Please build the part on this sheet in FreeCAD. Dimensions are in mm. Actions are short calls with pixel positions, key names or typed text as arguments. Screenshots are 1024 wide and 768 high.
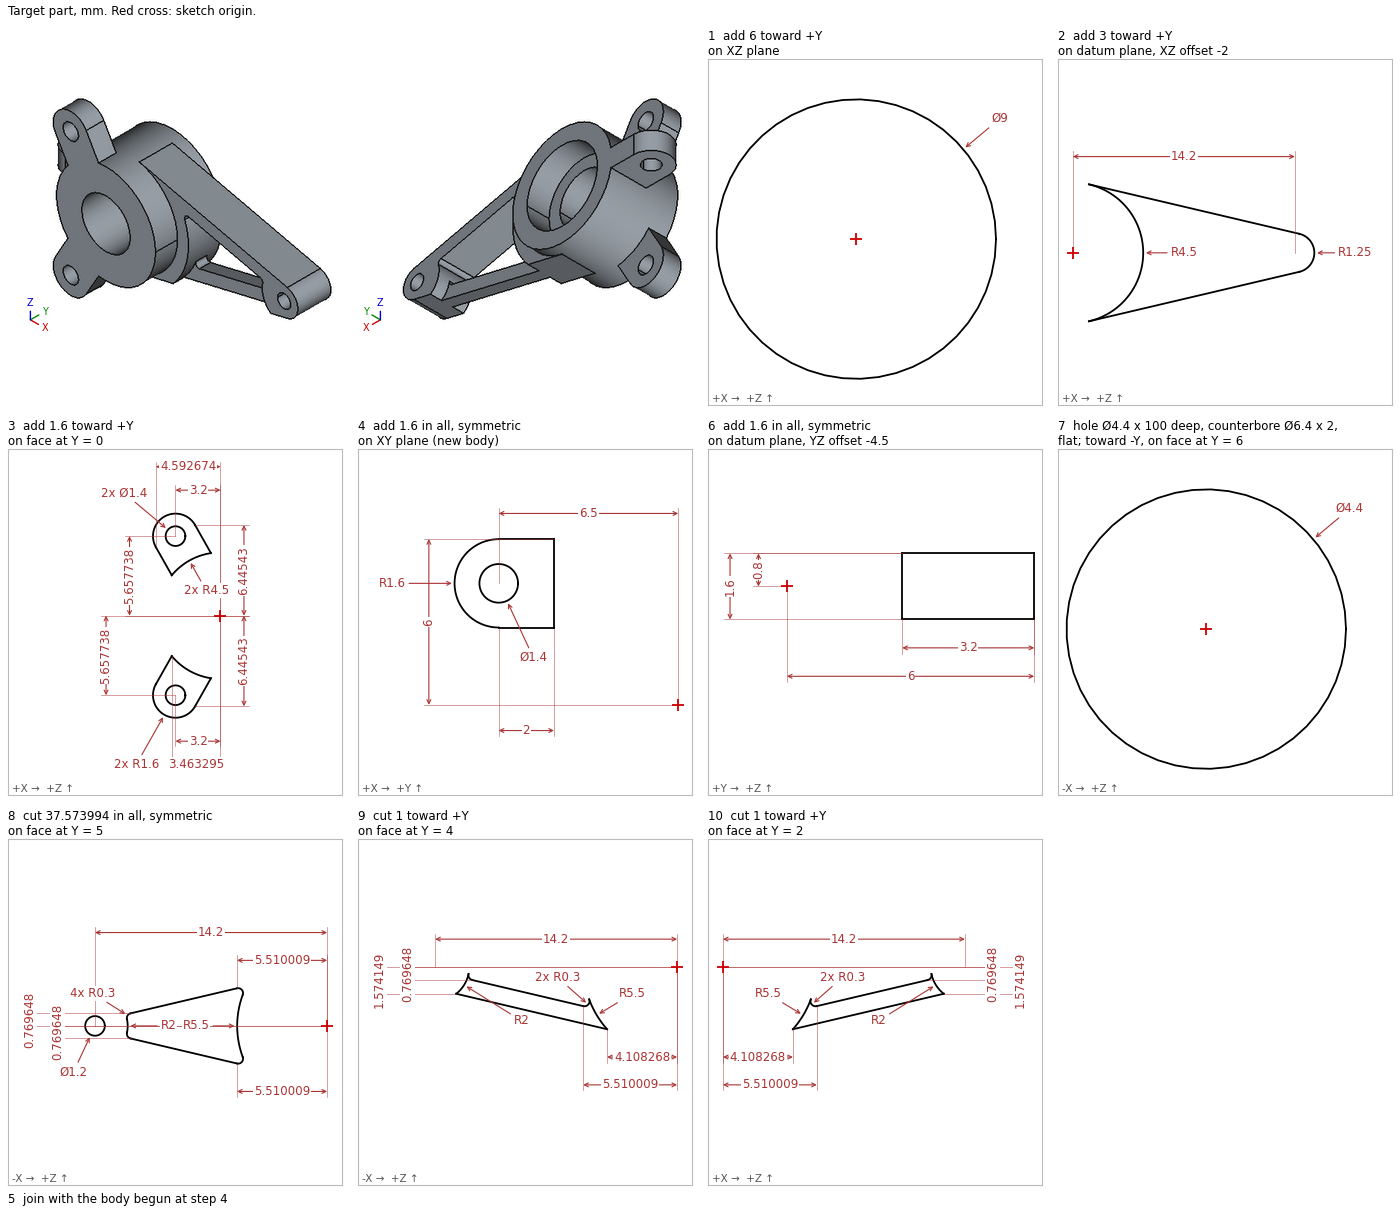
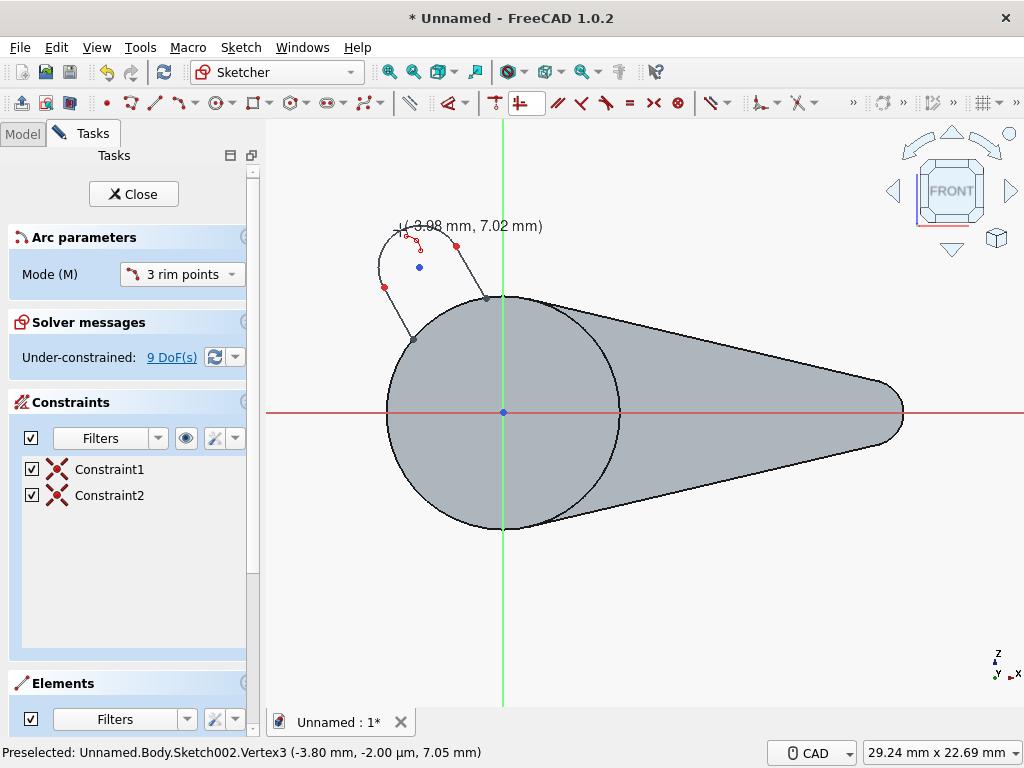
click(413, 340)
click(486, 299)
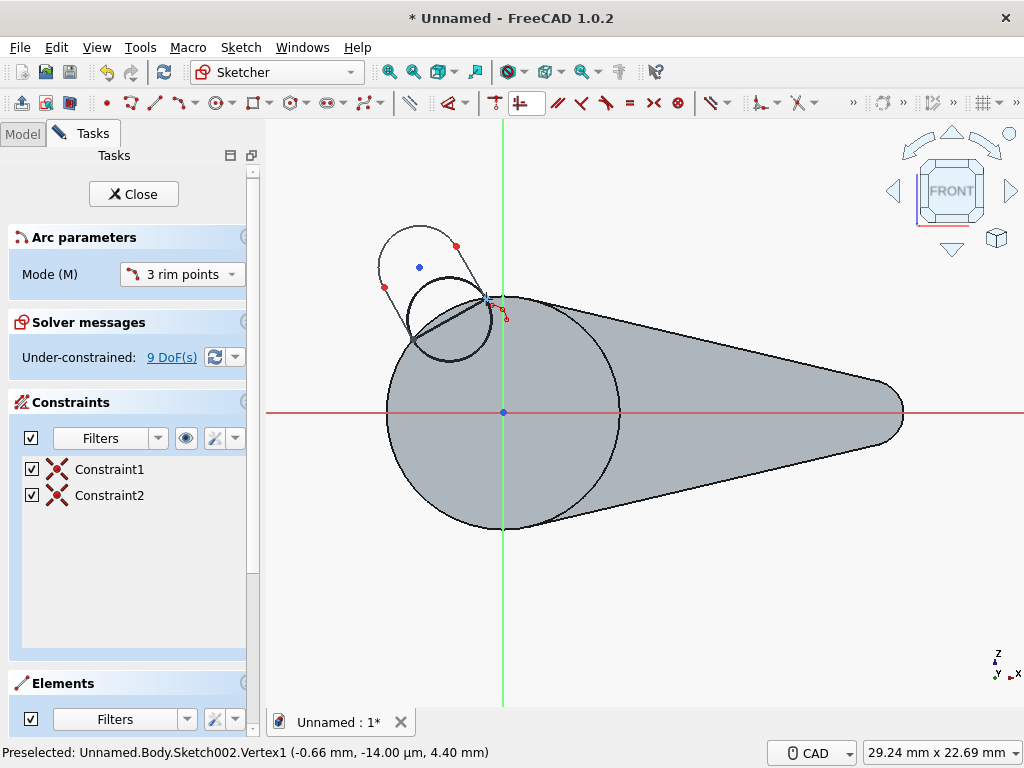
scroll(446, 311, up, 4)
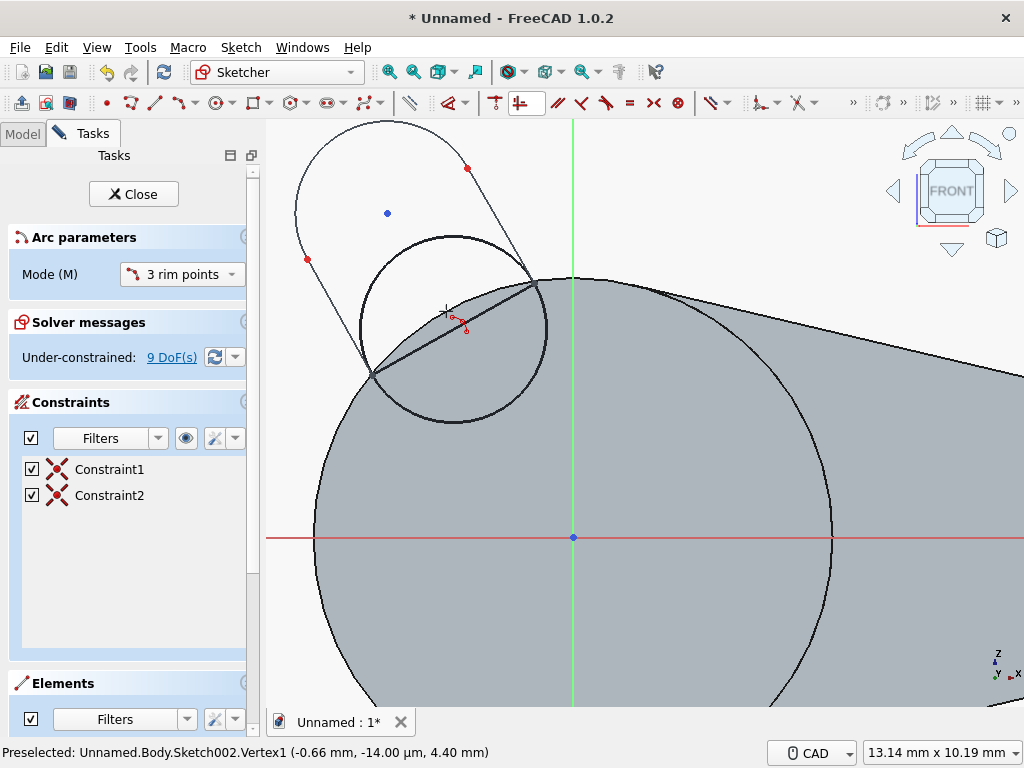
click(445, 312)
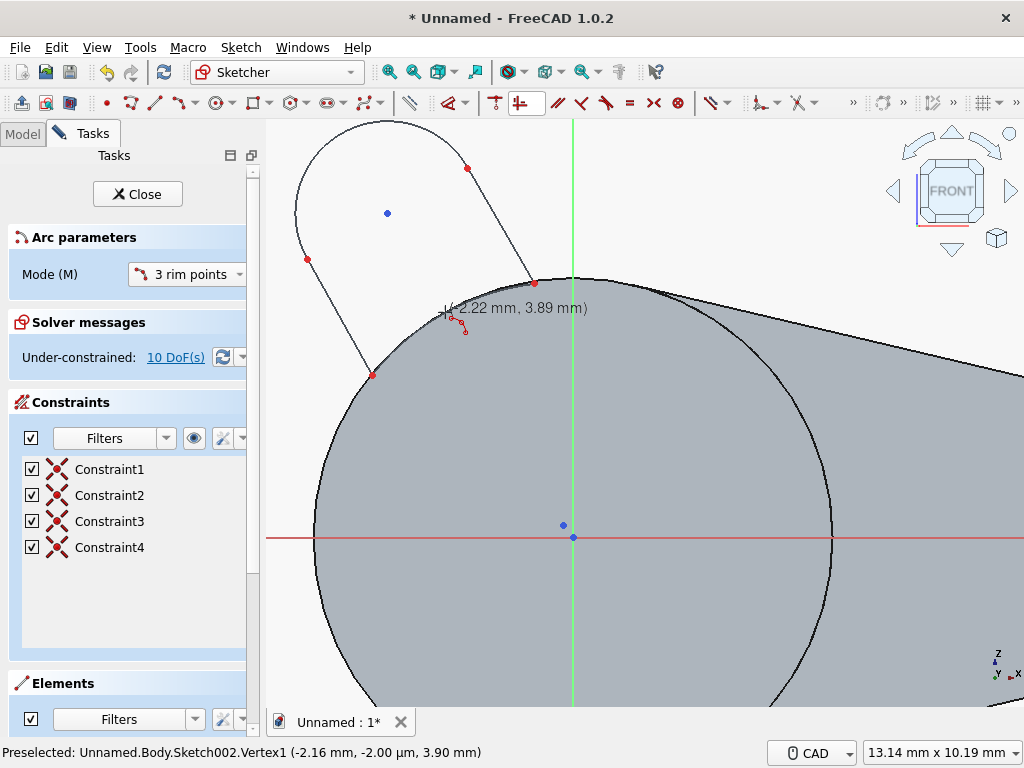
click(156, 104)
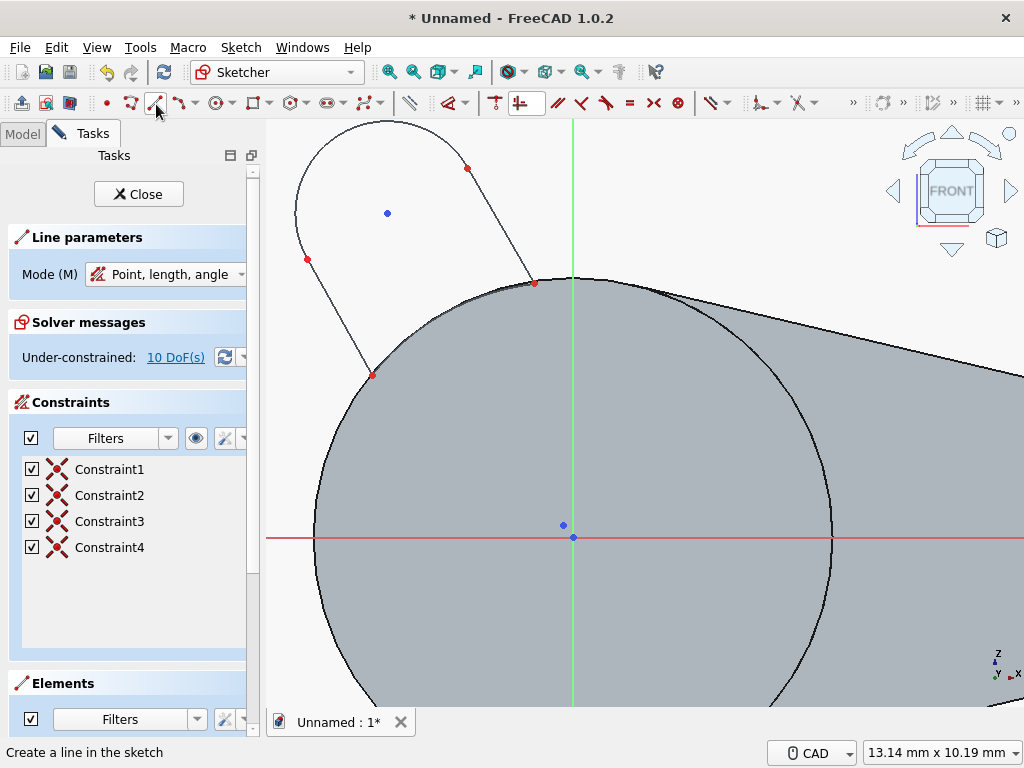
scroll(687, 311, down, 4)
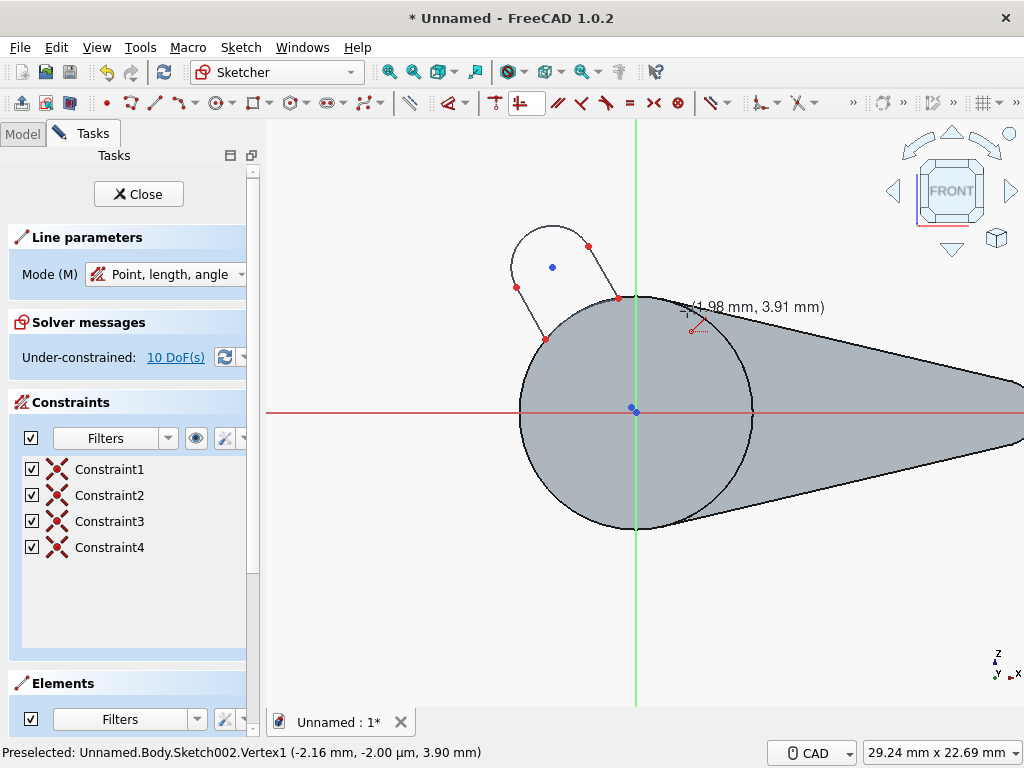
click(589, 580)
click(619, 528)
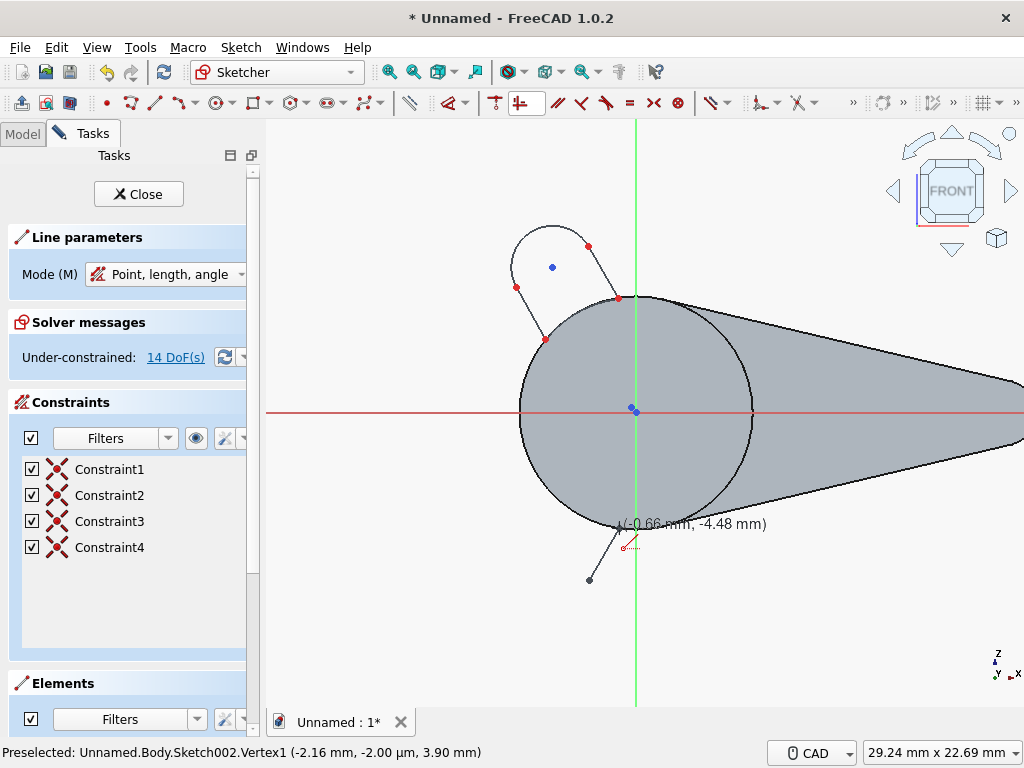
click(546, 487)
click(517, 539)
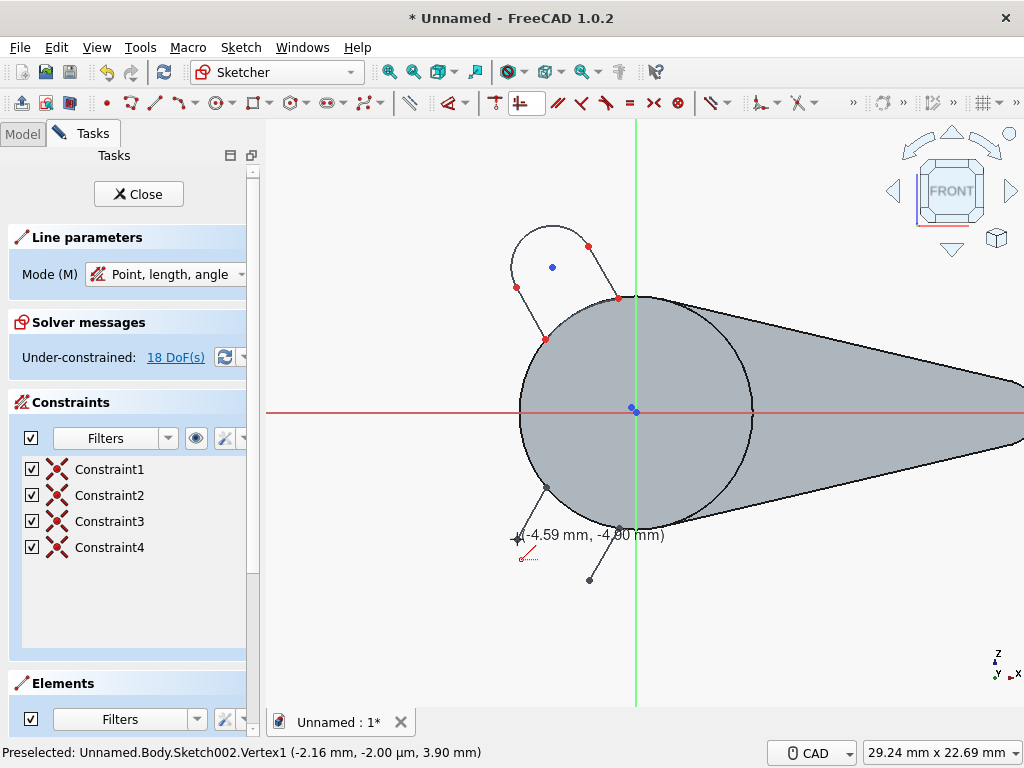
key(g)
key(3)
key(a)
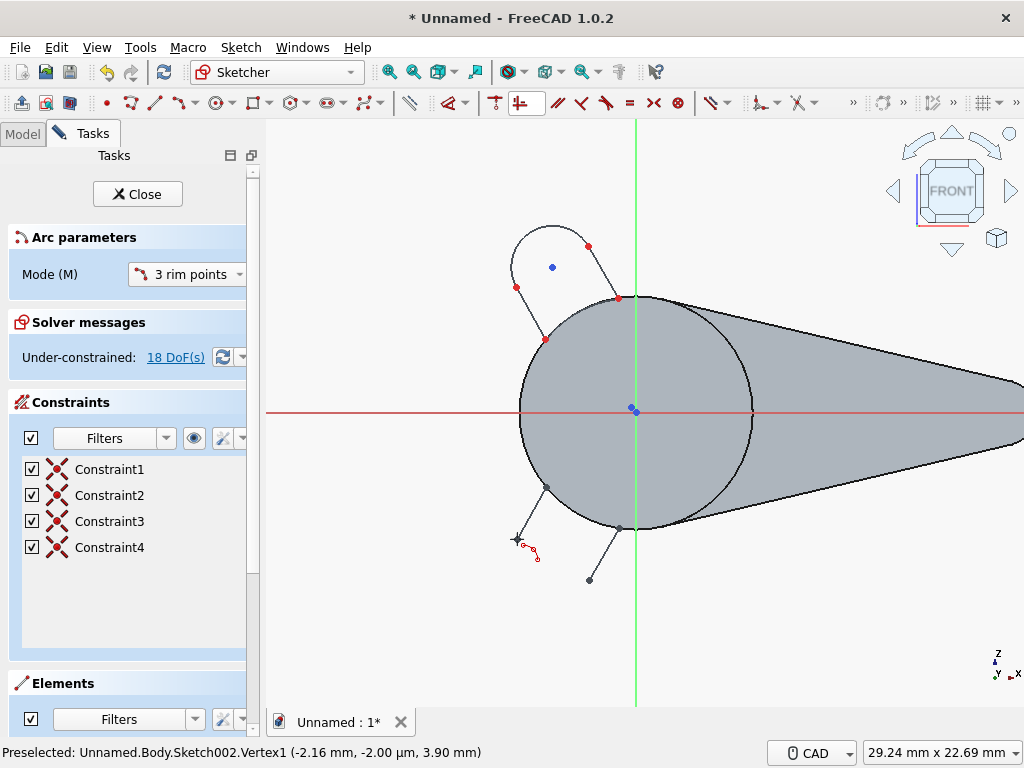
click(619, 529)
click(546, 488)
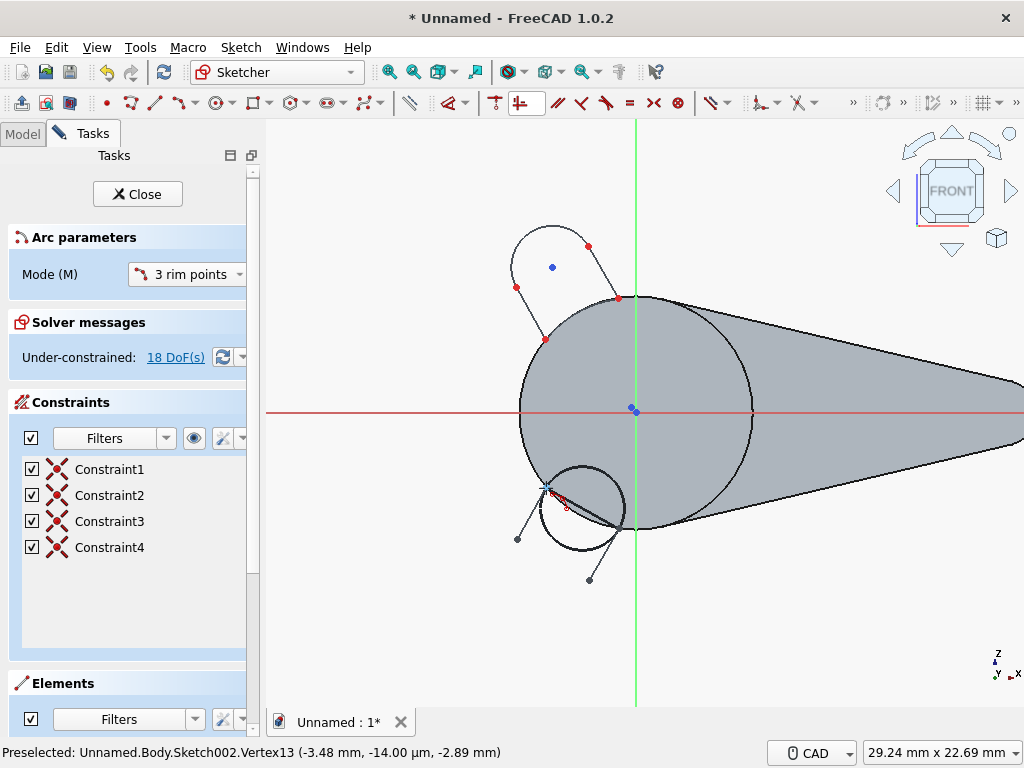
scroll(579, 515, up, 4)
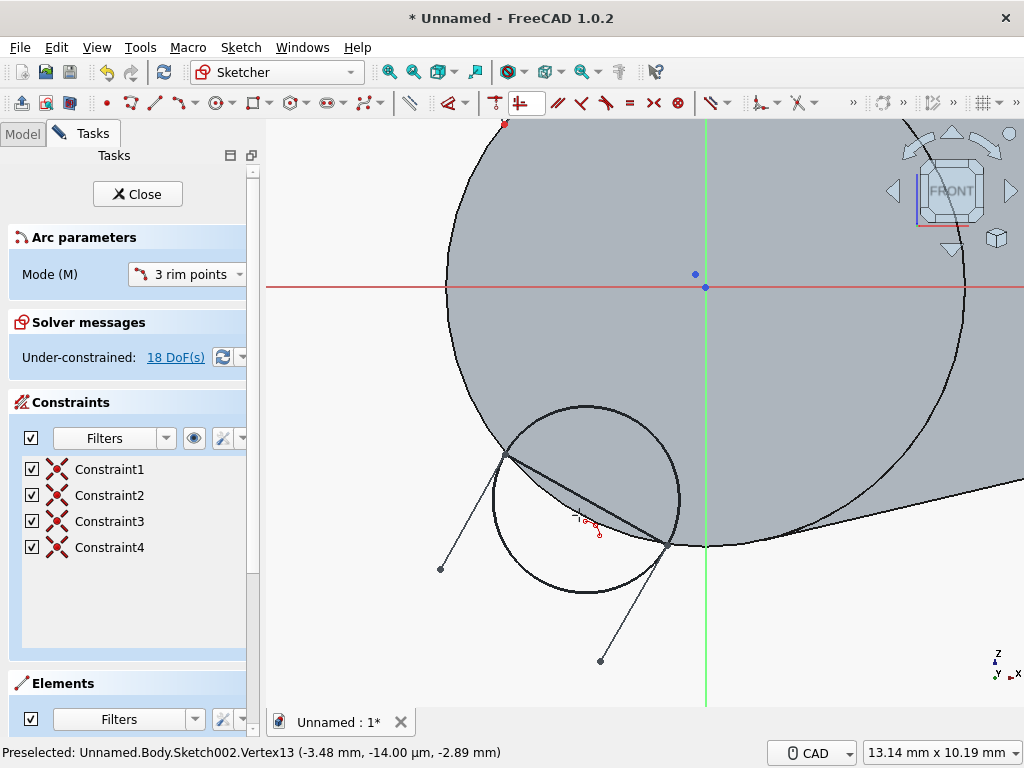
click(578, 513)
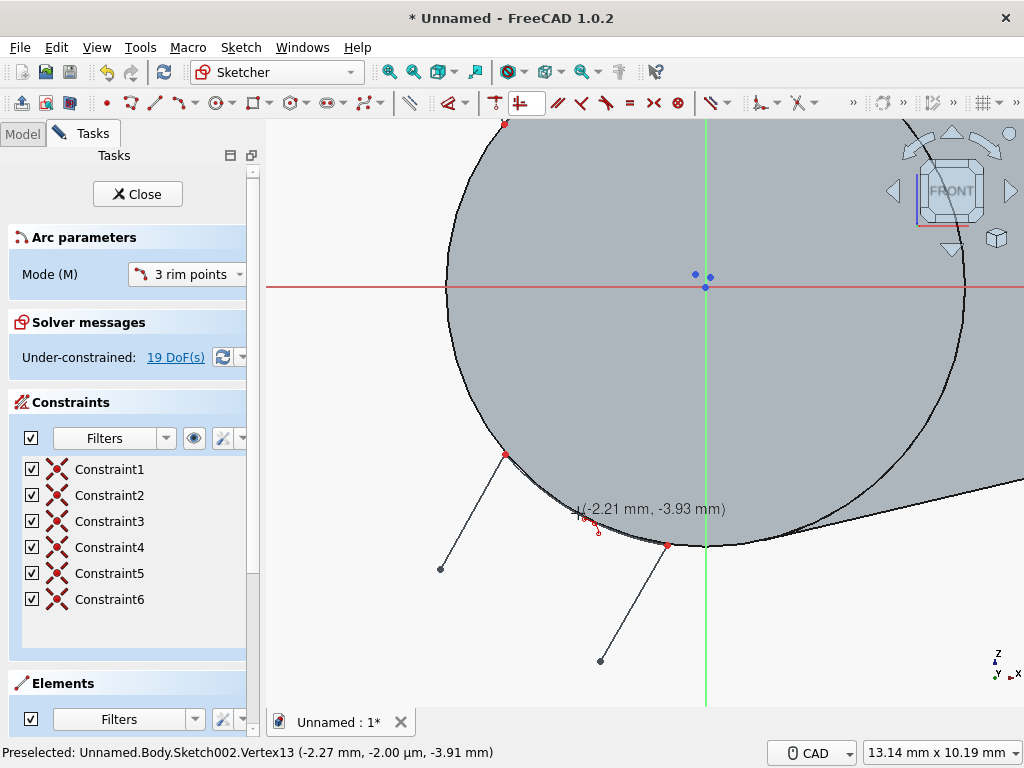
click(441, 570)
click(601, 661)